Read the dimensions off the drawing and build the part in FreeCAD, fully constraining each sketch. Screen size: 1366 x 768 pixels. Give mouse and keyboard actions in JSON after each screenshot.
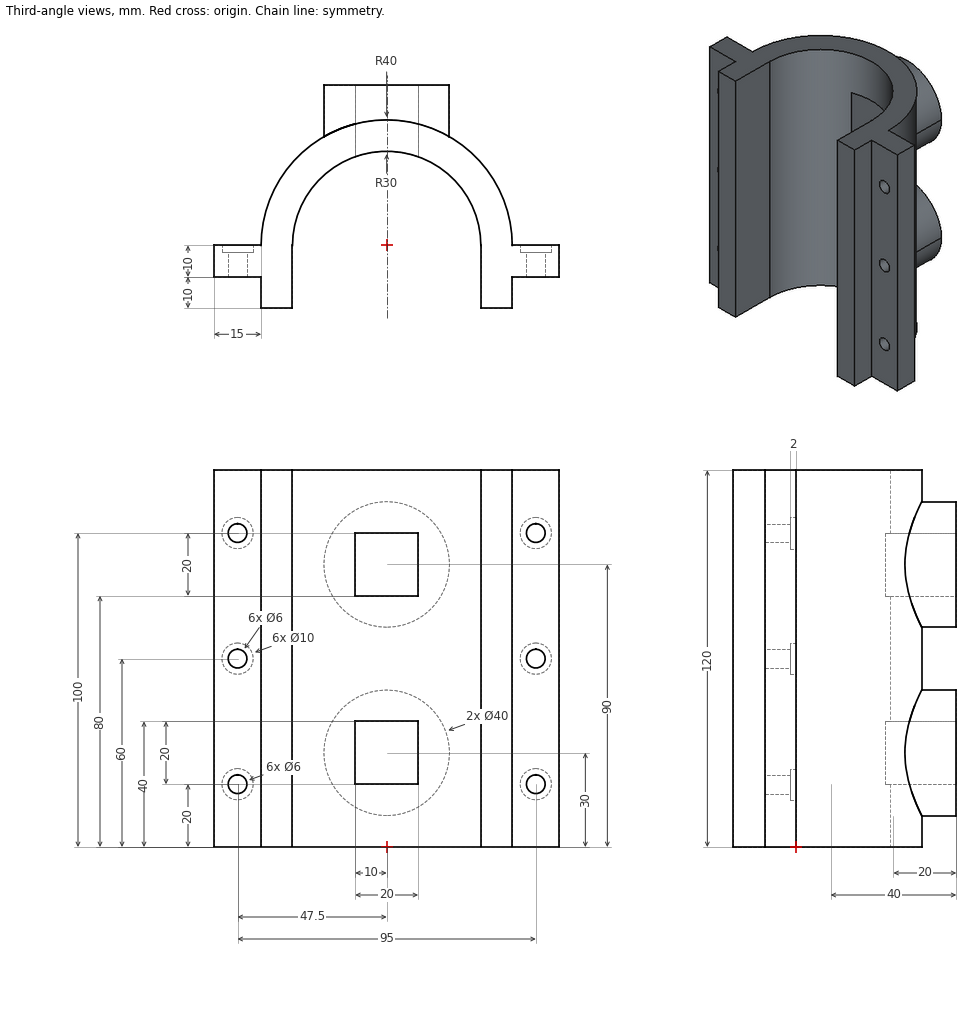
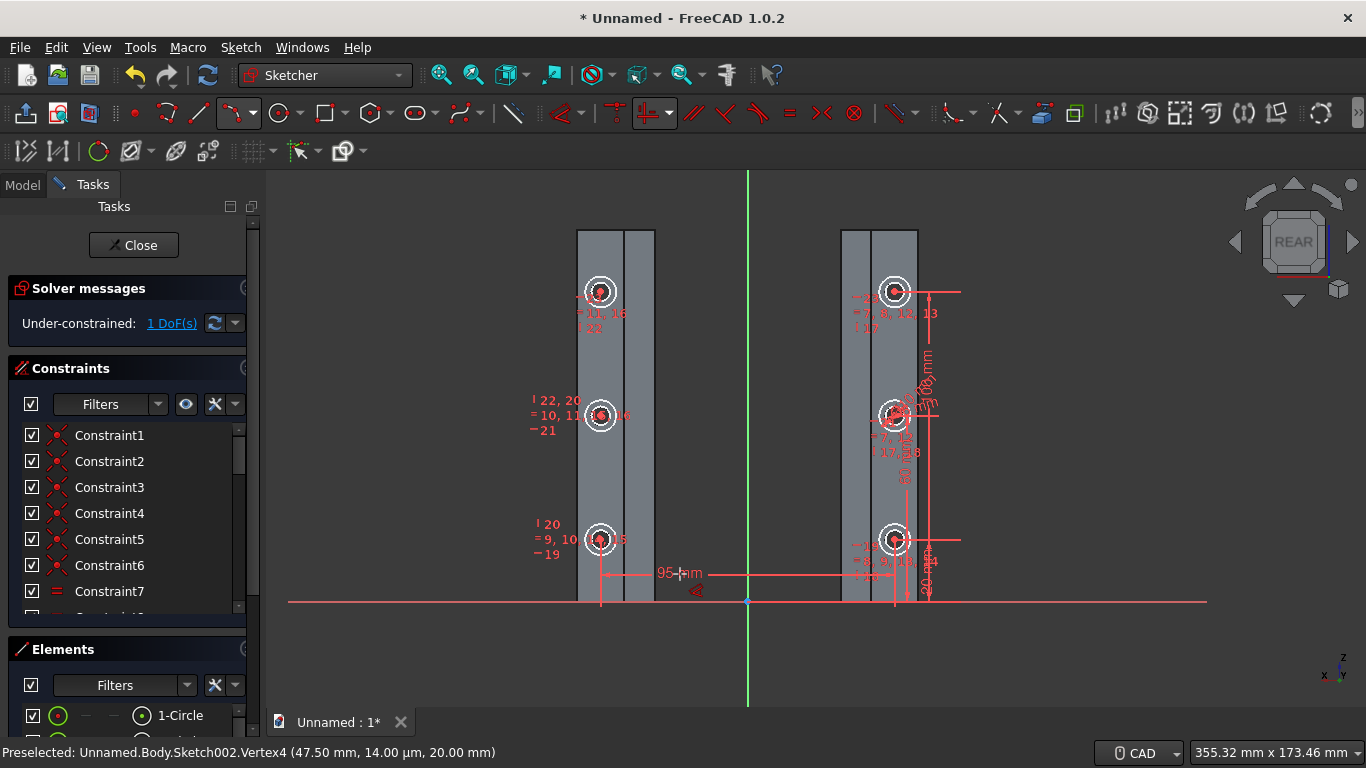
{"action": "left_click", "coordinate": [895, 416]}
{"action": "left_click", "coordinate": [821, 636]}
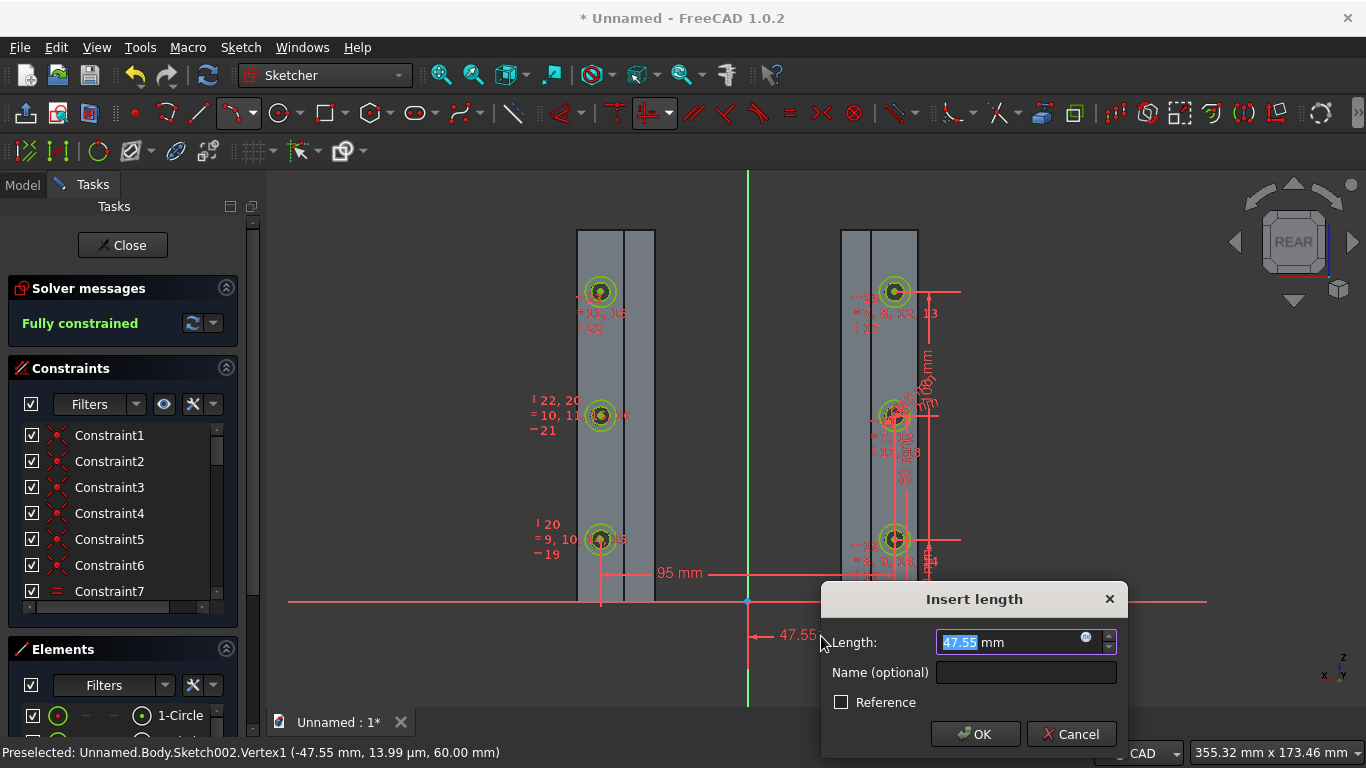
{"action": "type", "text": "47.5"}
{"action": "key", "text": "Return"}
{"action": "key", "text": "Escape"}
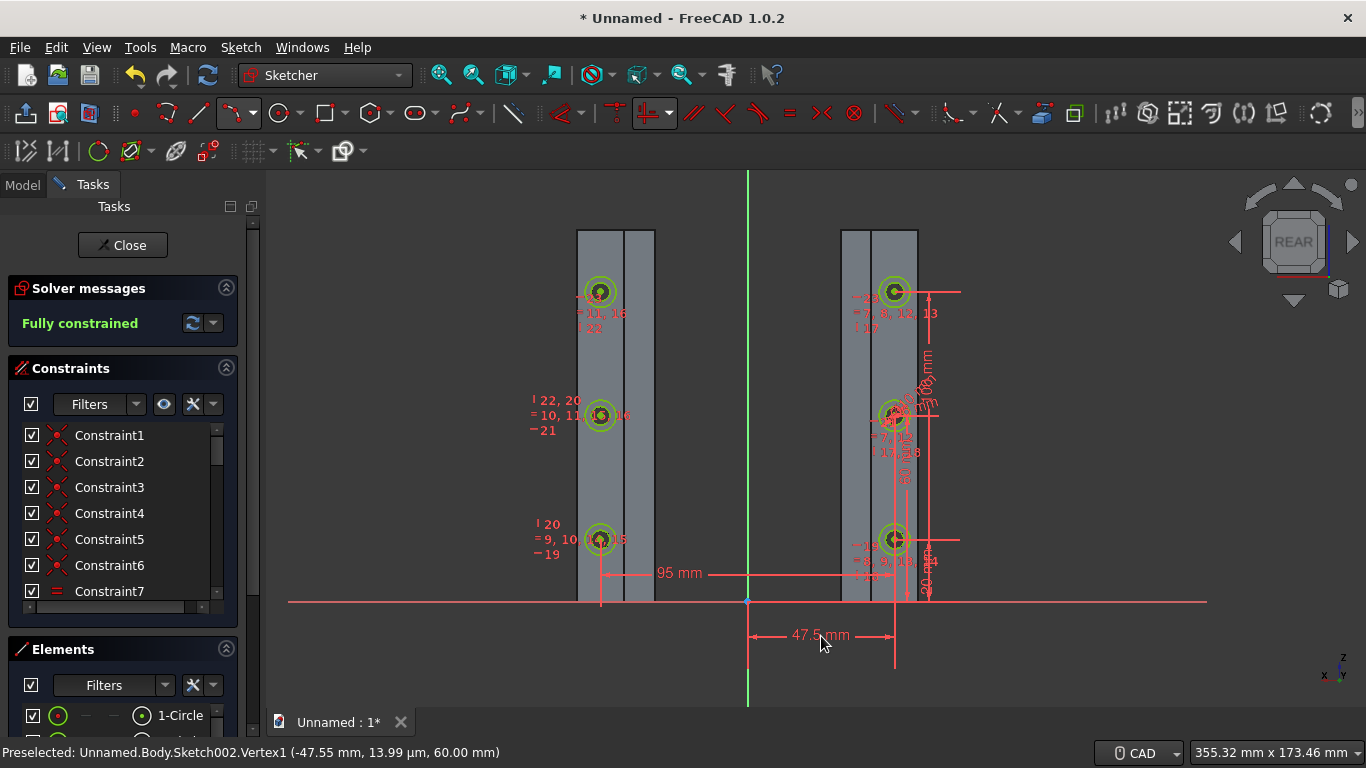
{"action": "left_click", "coordinate": [123, 245]}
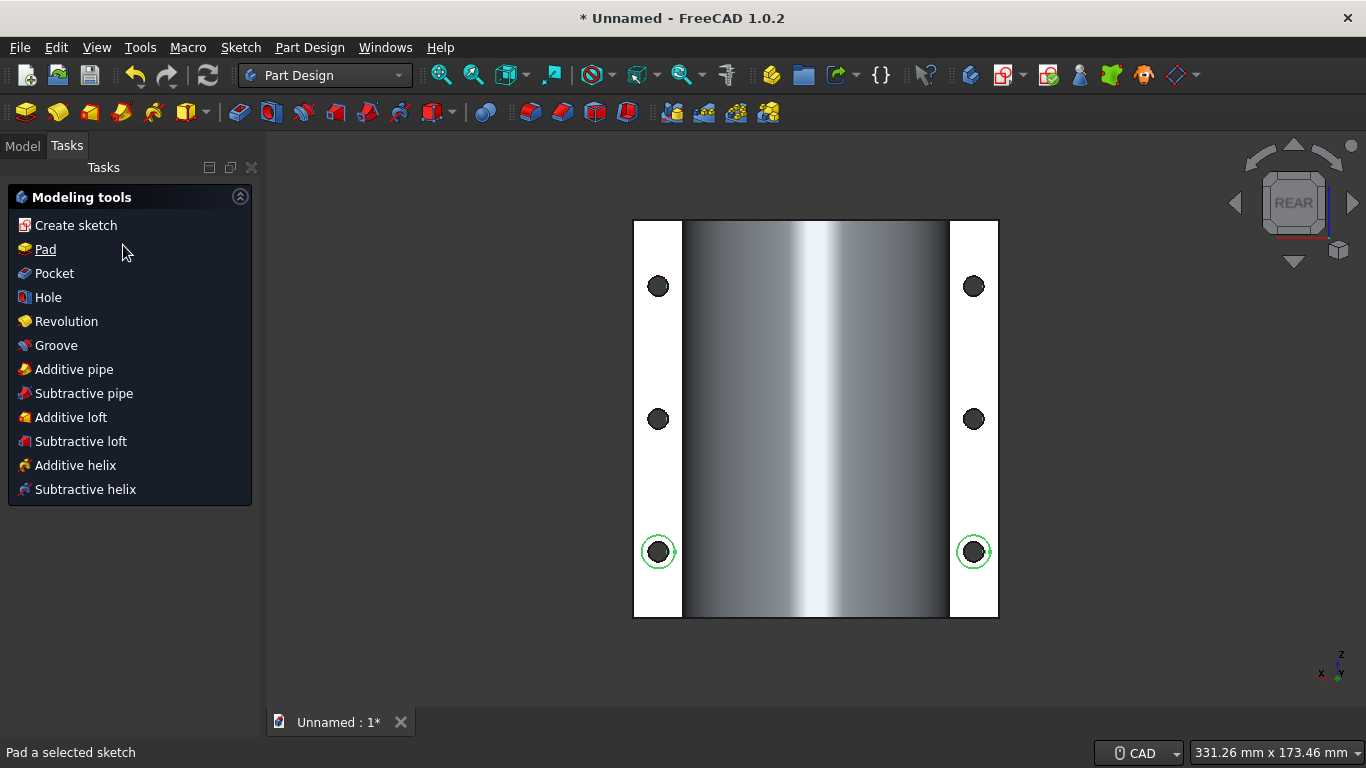
{"action": "left_click", "coordinate": [240, 112]}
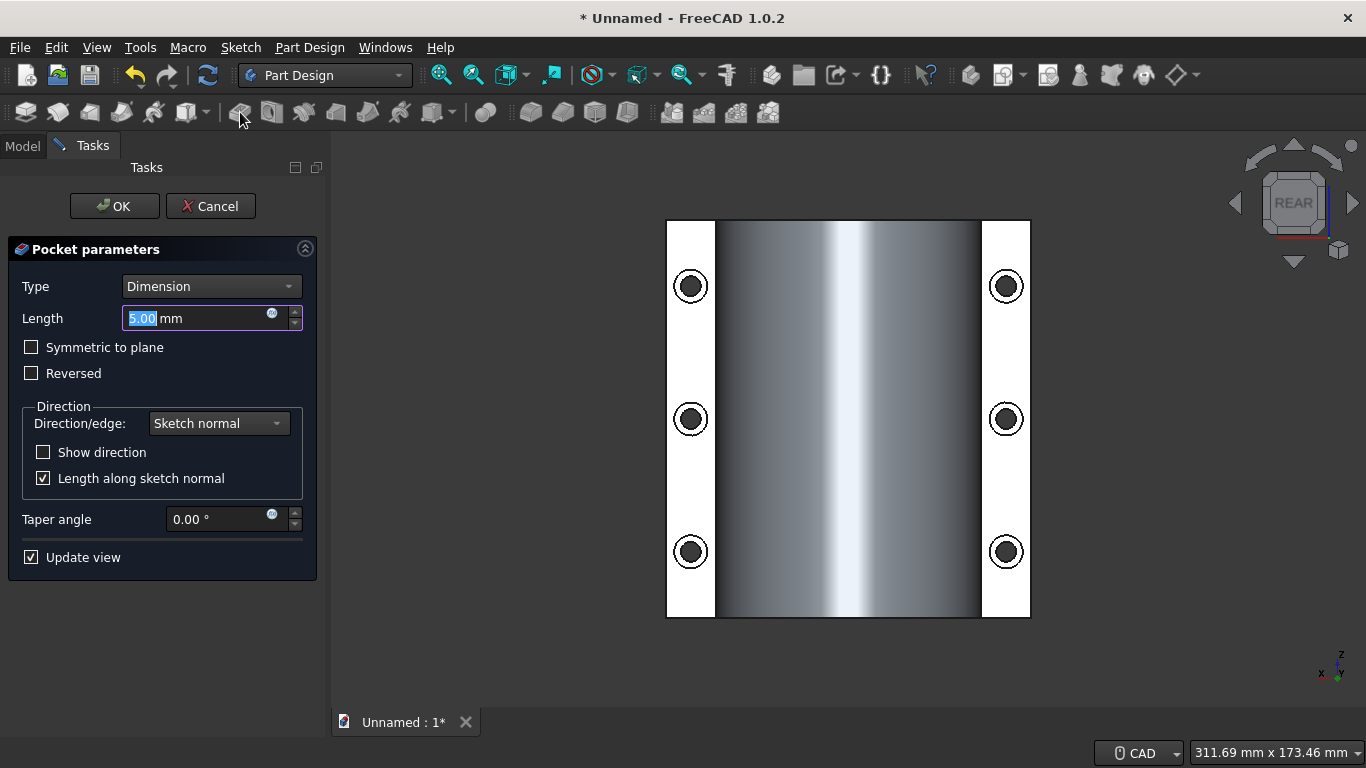
{"action": "type", "text": "2"}
{"action": "key", "text": "Tab"}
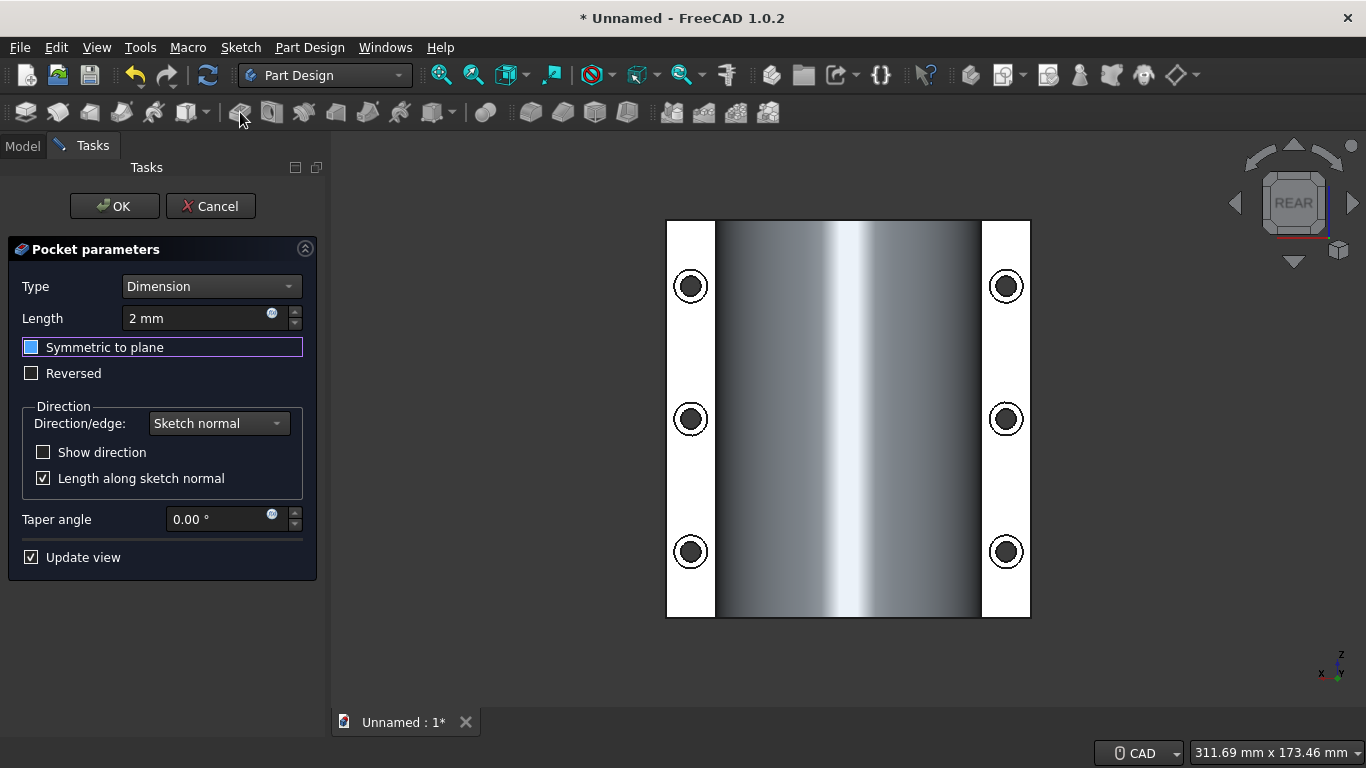
{"action": "left_click", "coordinate": [115, 206]}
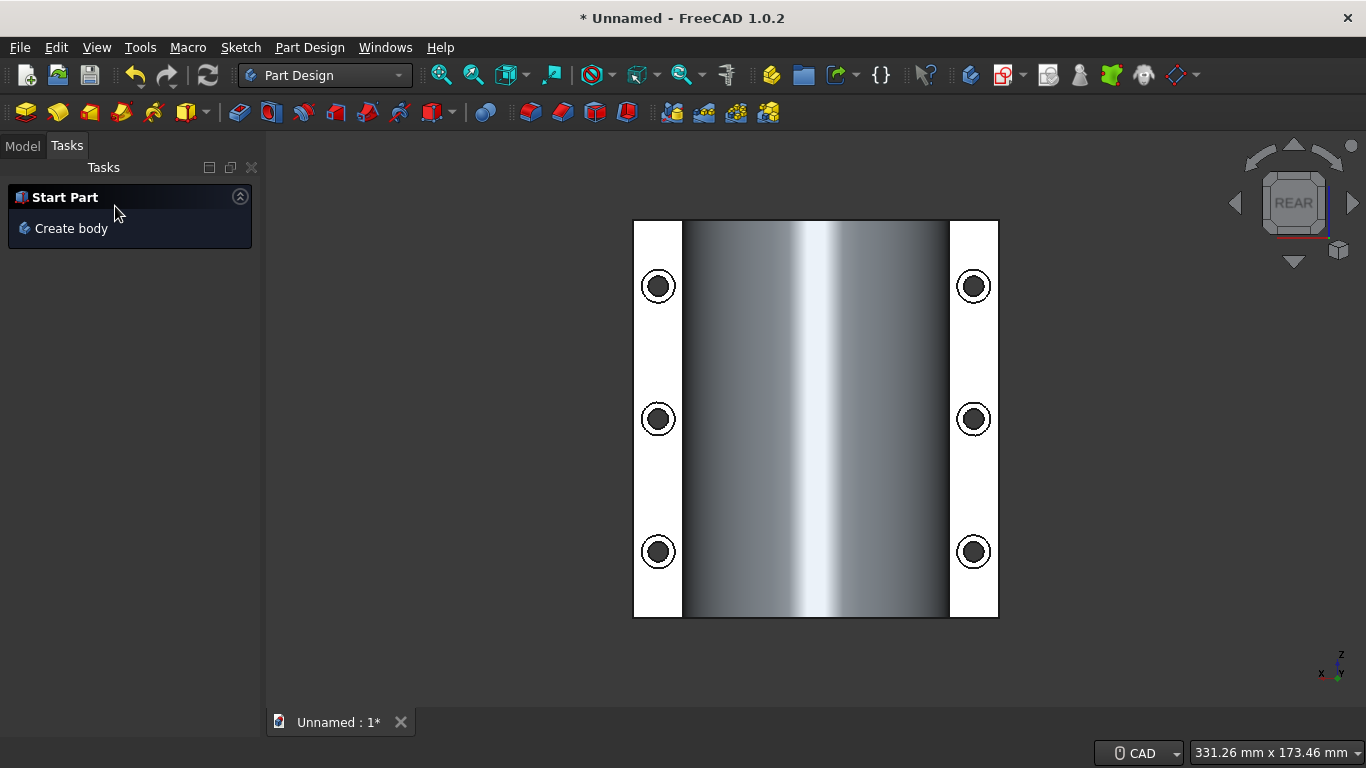
{"action": "left_click", "coordinate": [23, 145]}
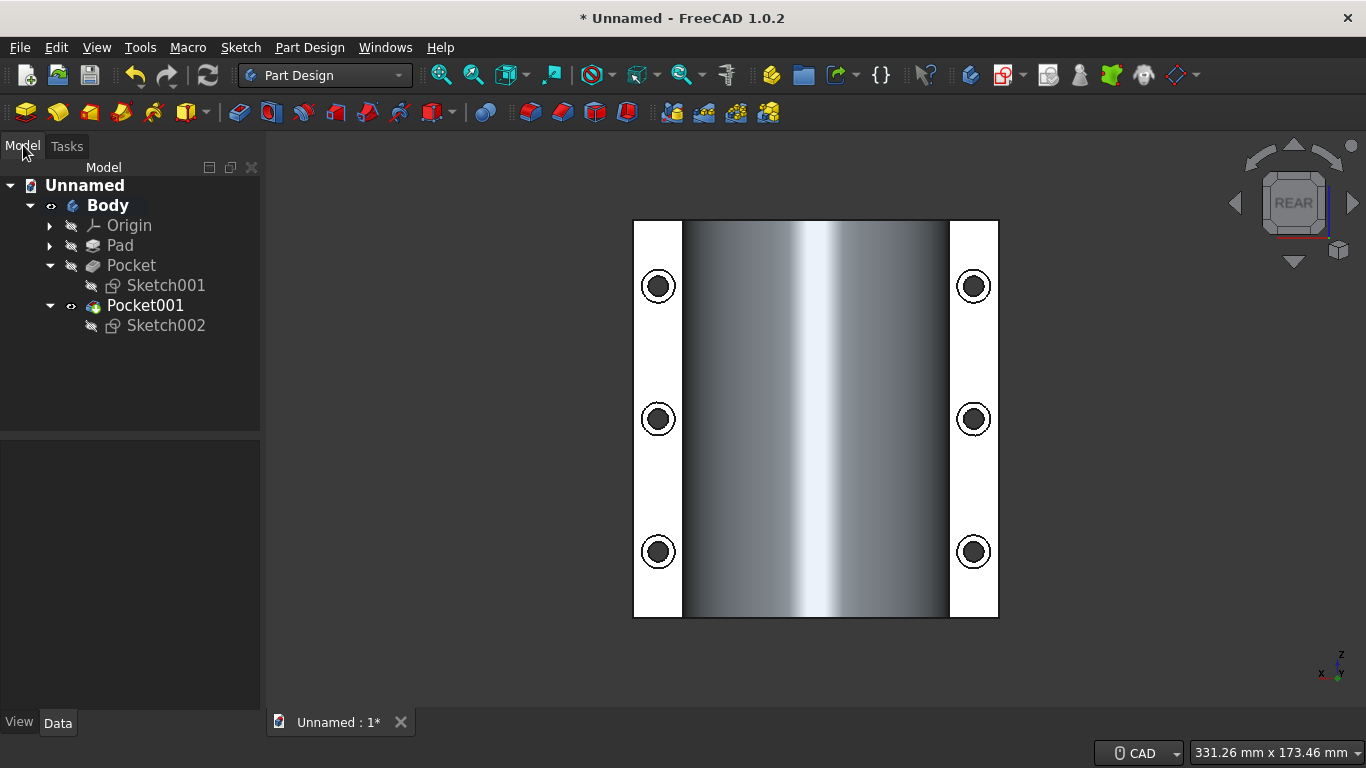
{"action": "left_click", "coordinate": [50, 226]}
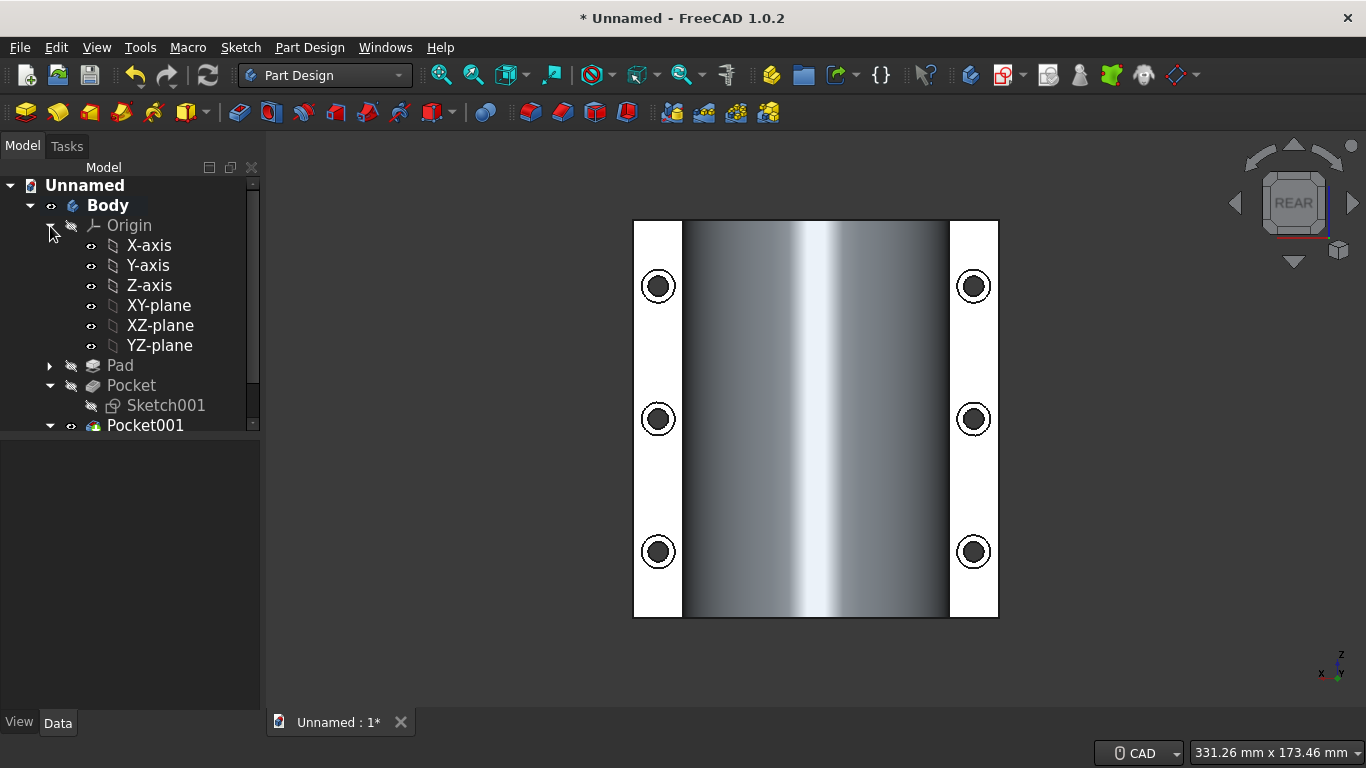
{"action": "left_click", "coordinate": [136, 326]}